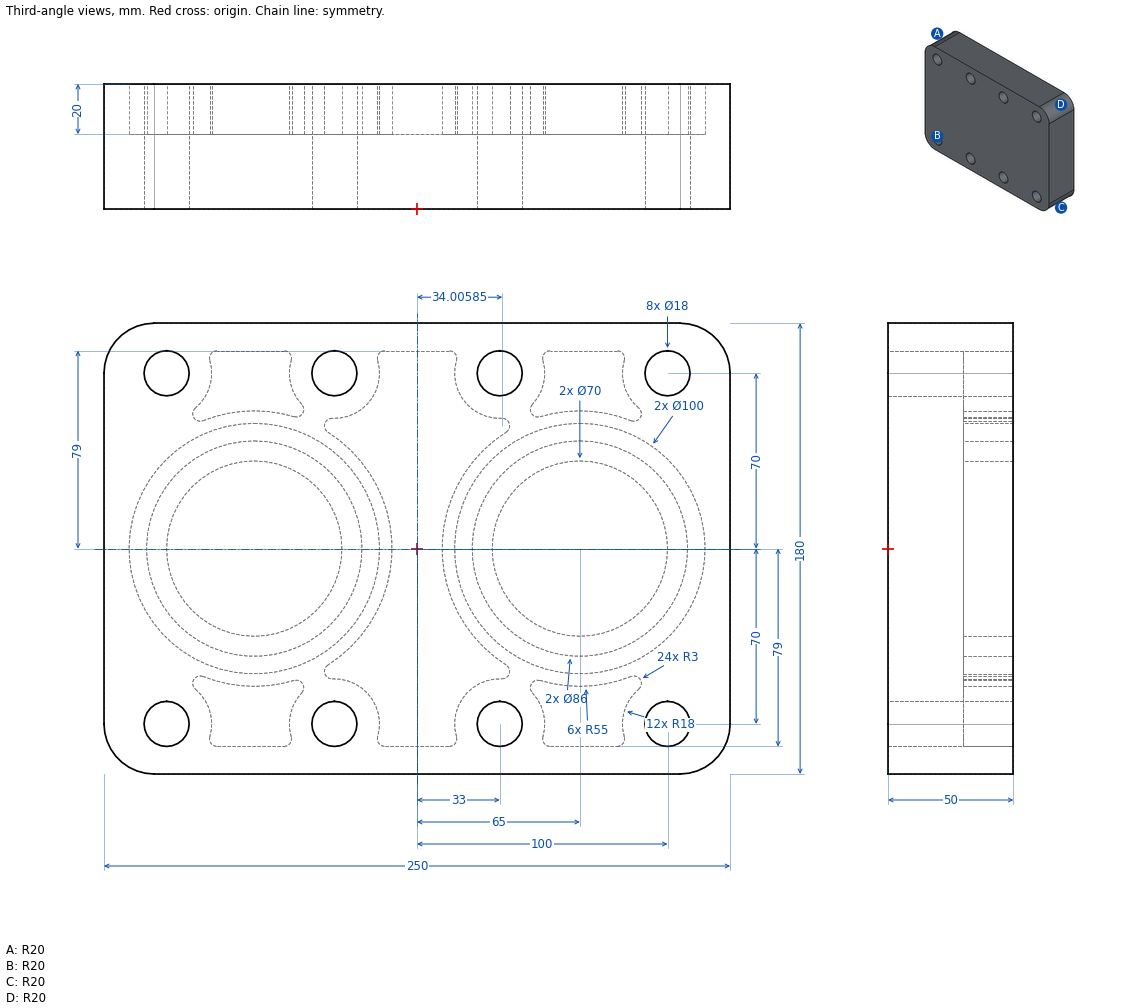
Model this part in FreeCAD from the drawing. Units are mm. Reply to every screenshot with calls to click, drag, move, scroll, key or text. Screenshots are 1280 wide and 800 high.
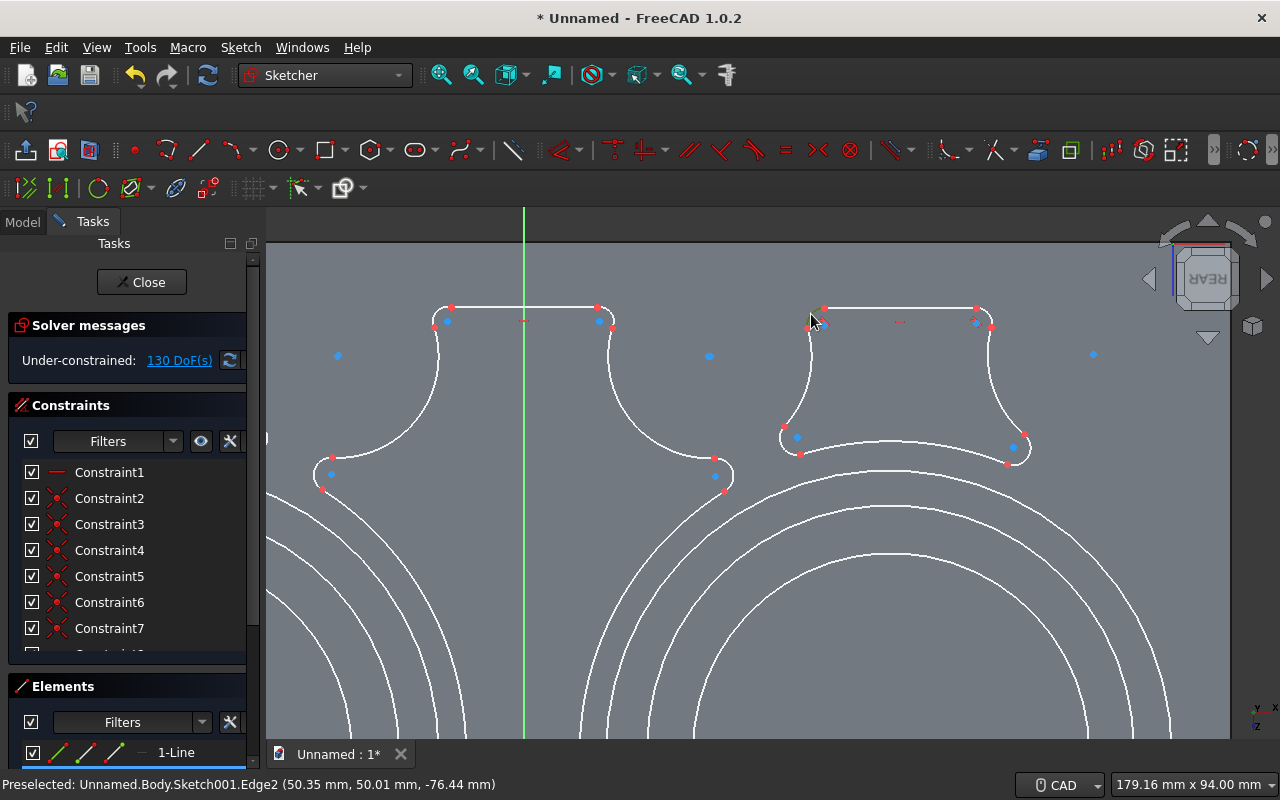
click(802, 401)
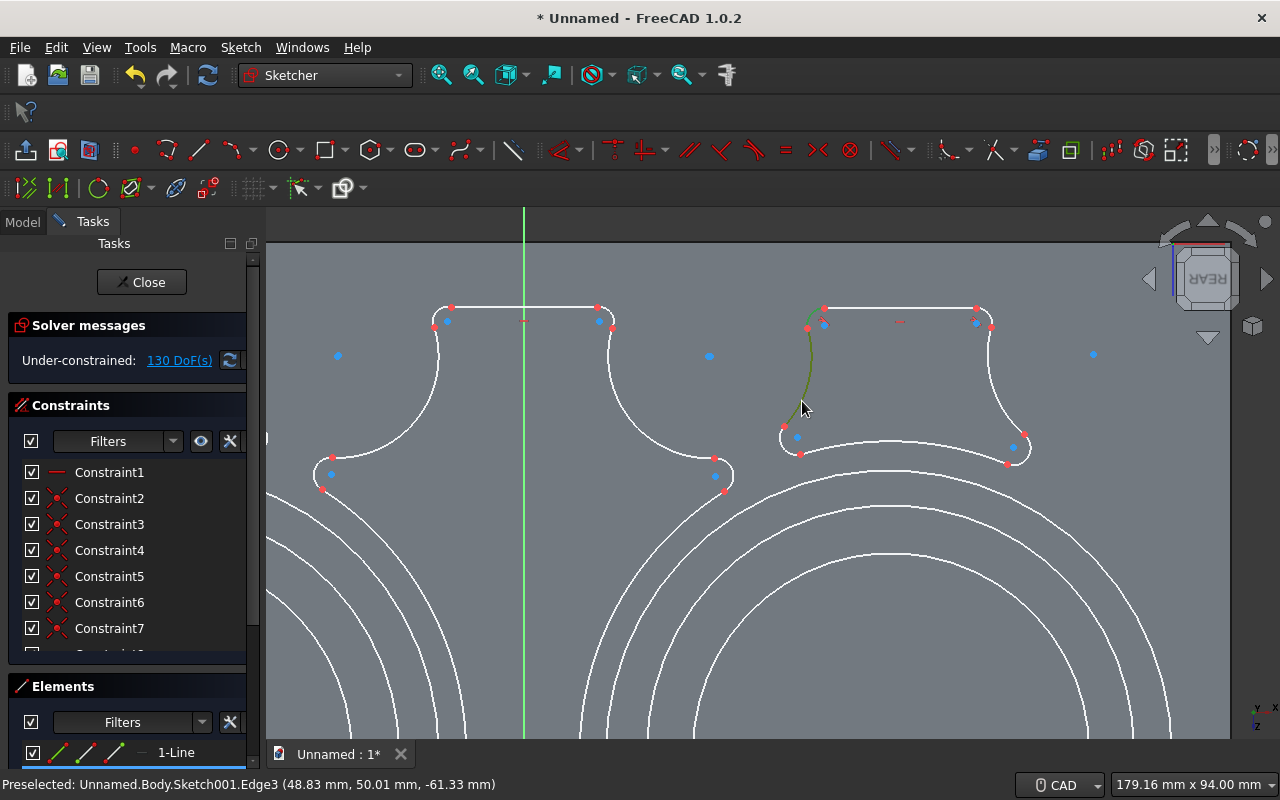
click(754, 150)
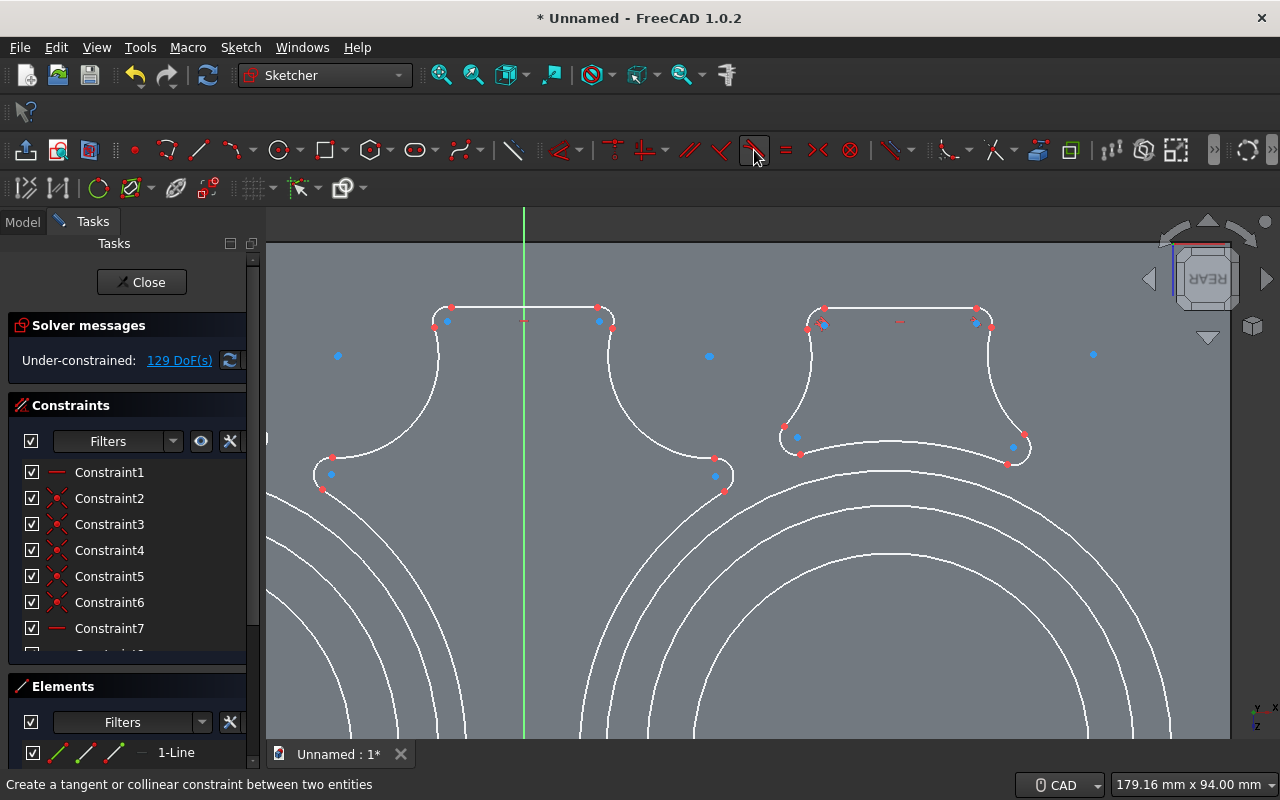
click(802, 401)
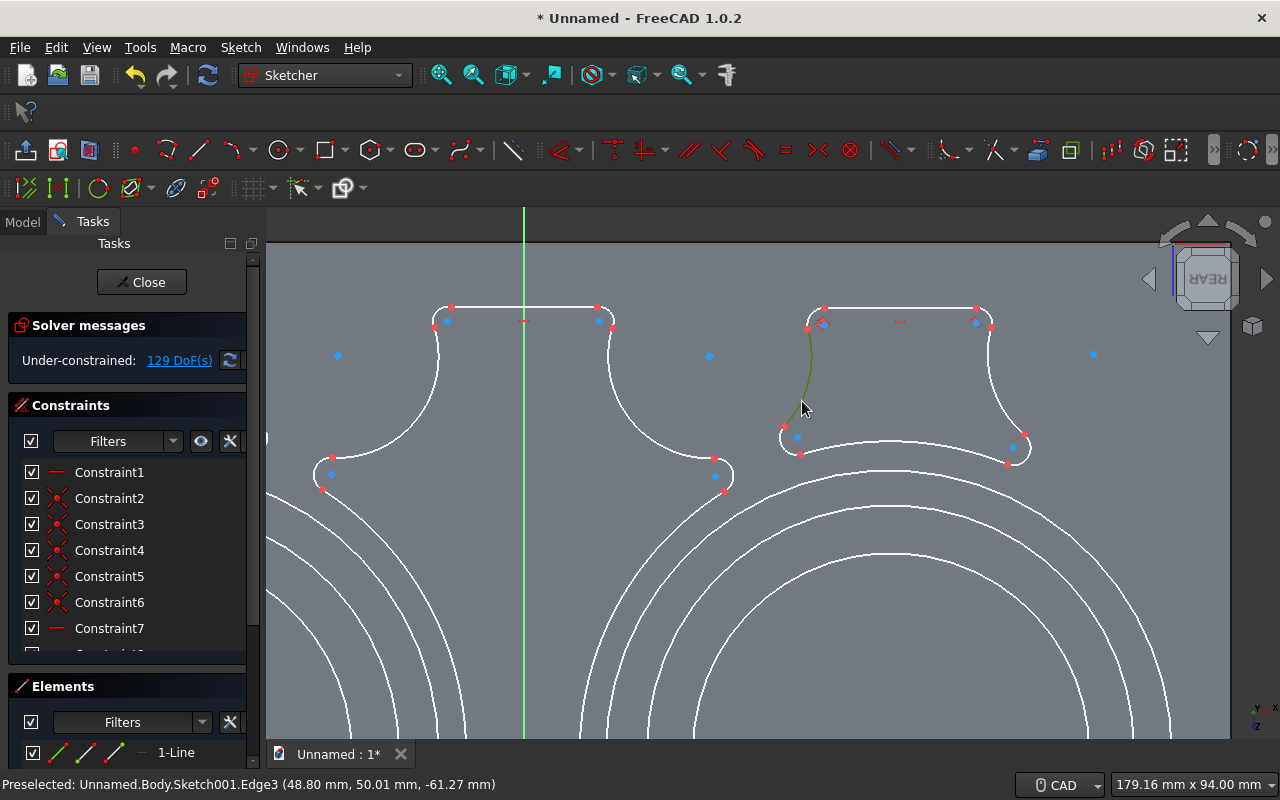
click(780, 439)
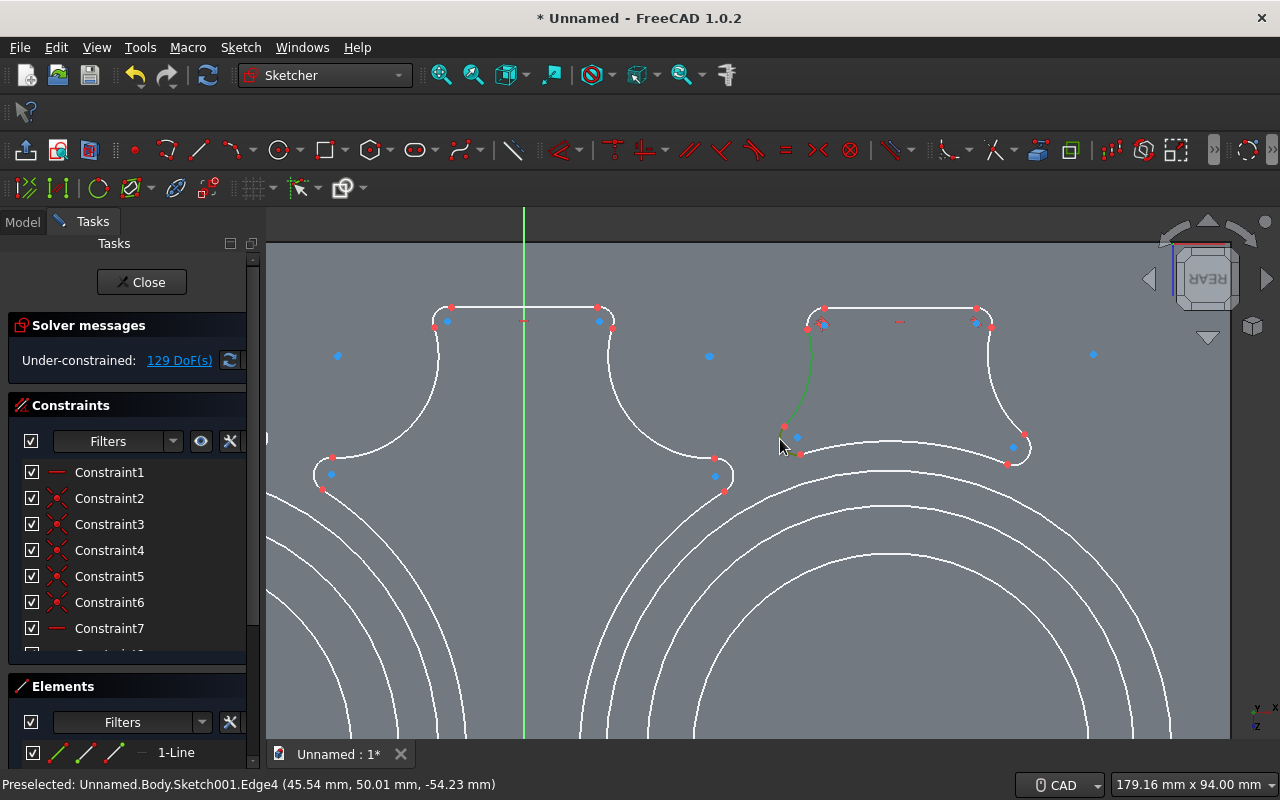
click(754, 150)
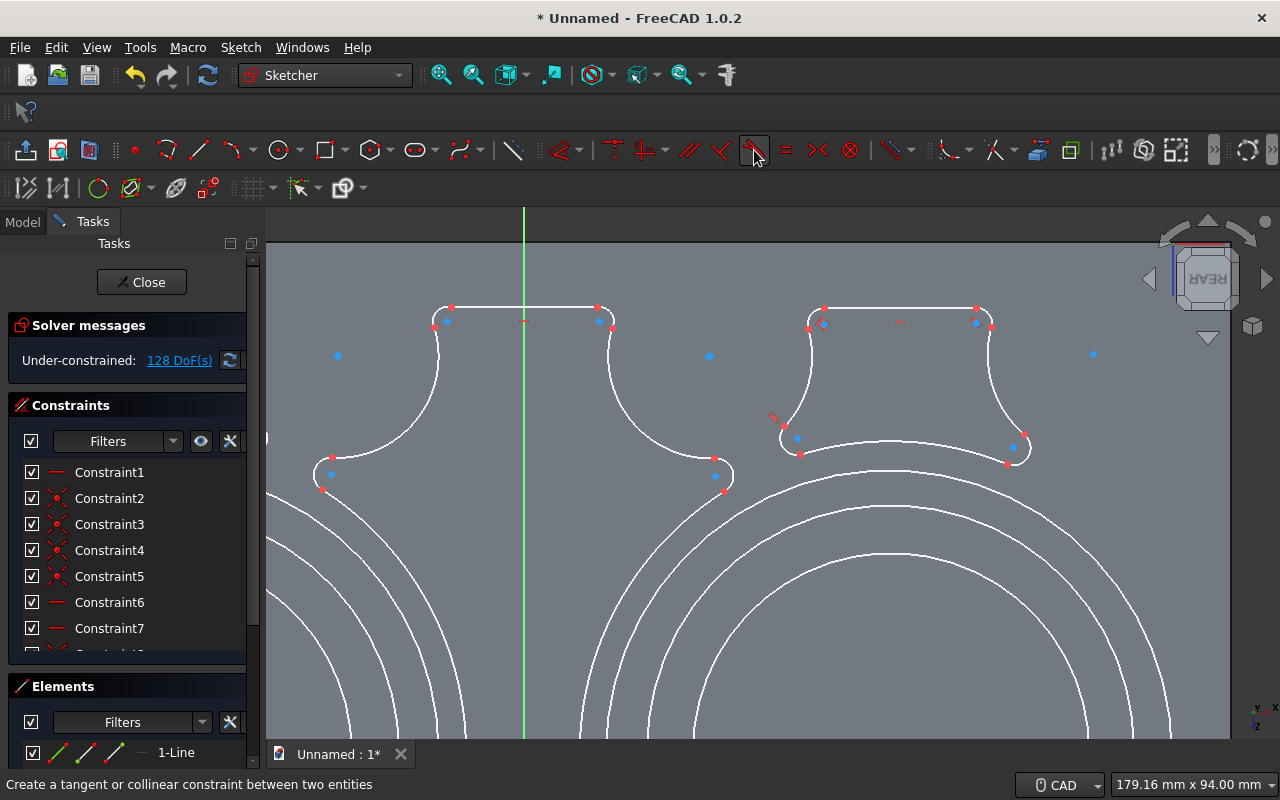
click(780, 438)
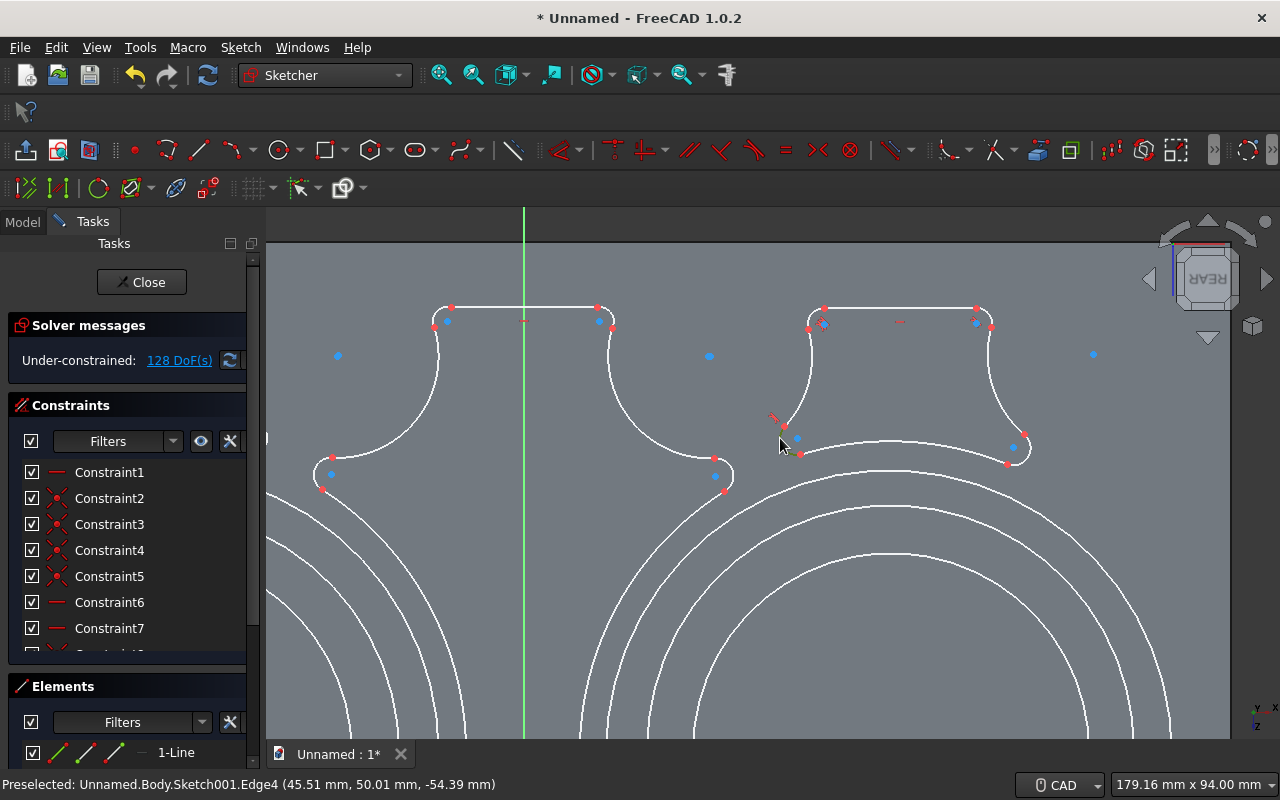
click(947, 447)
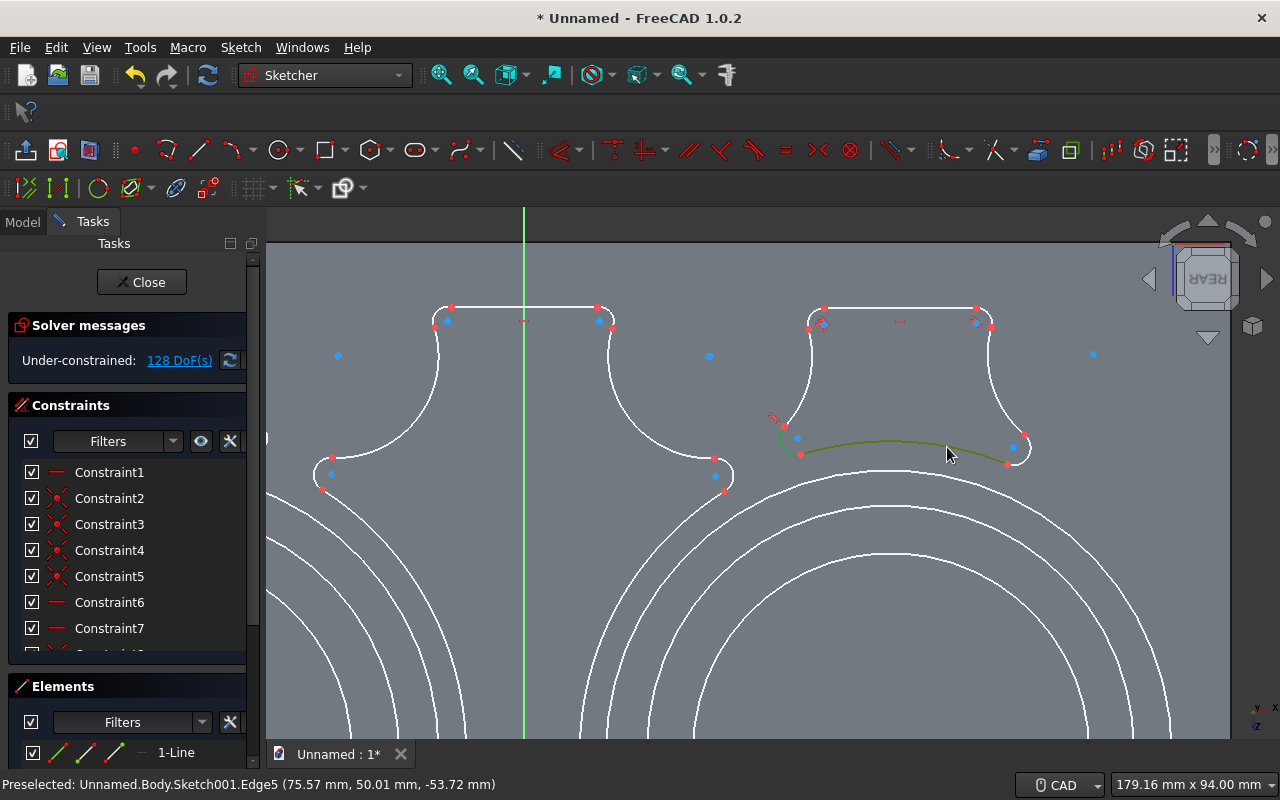
click(754, 150)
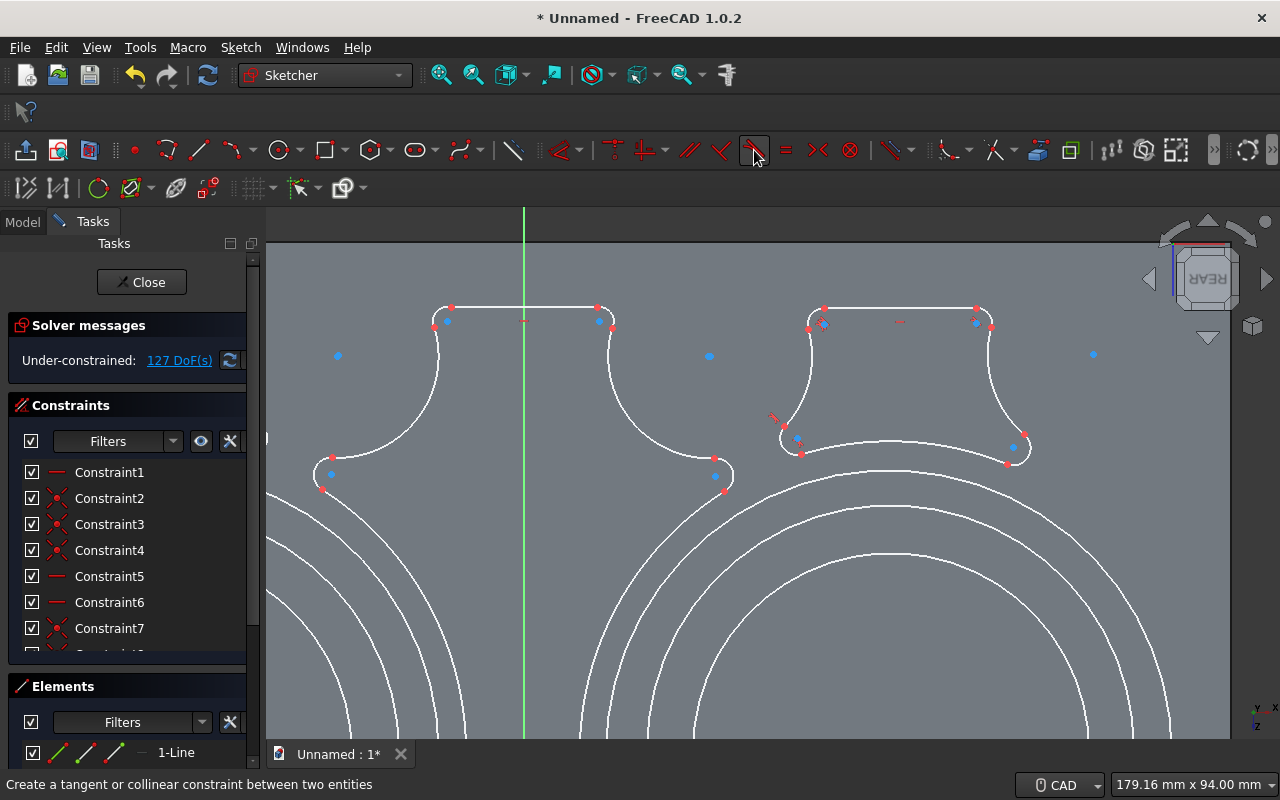
click(947, 447)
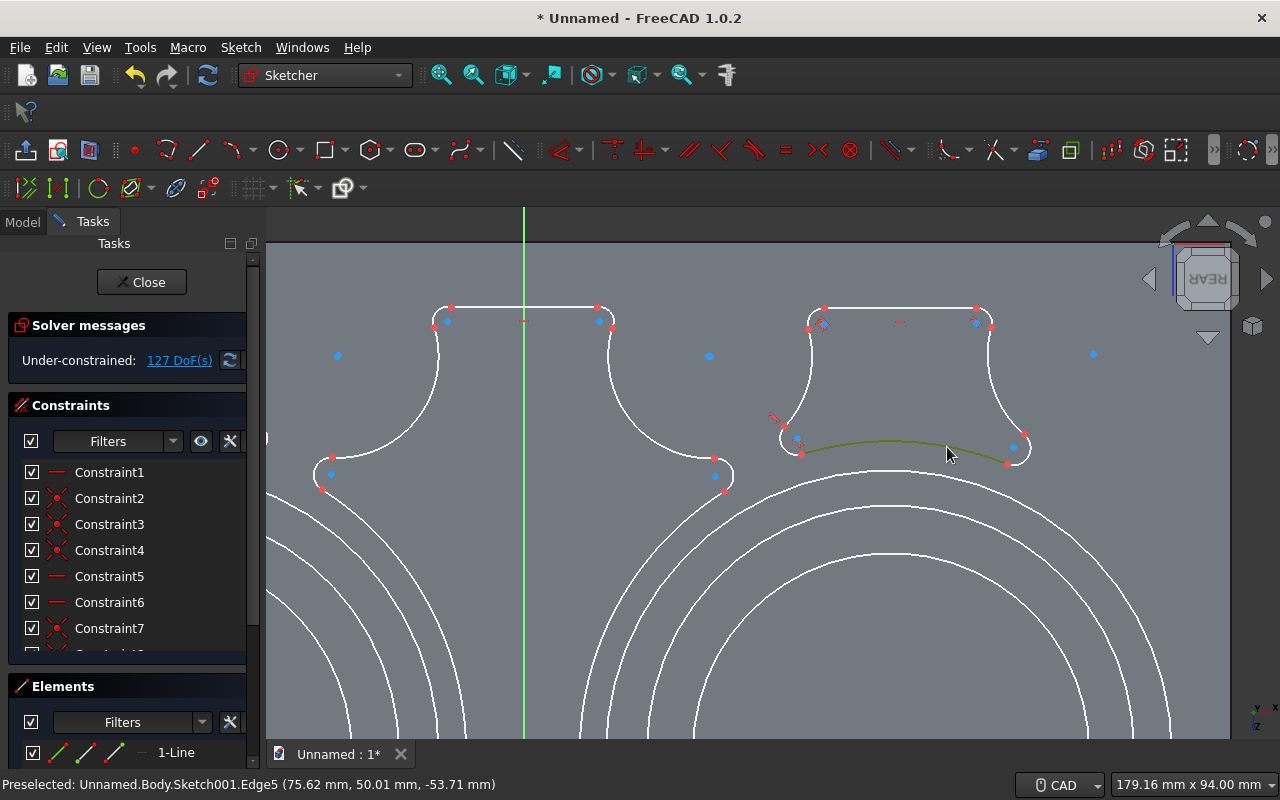
click(1022, 463)